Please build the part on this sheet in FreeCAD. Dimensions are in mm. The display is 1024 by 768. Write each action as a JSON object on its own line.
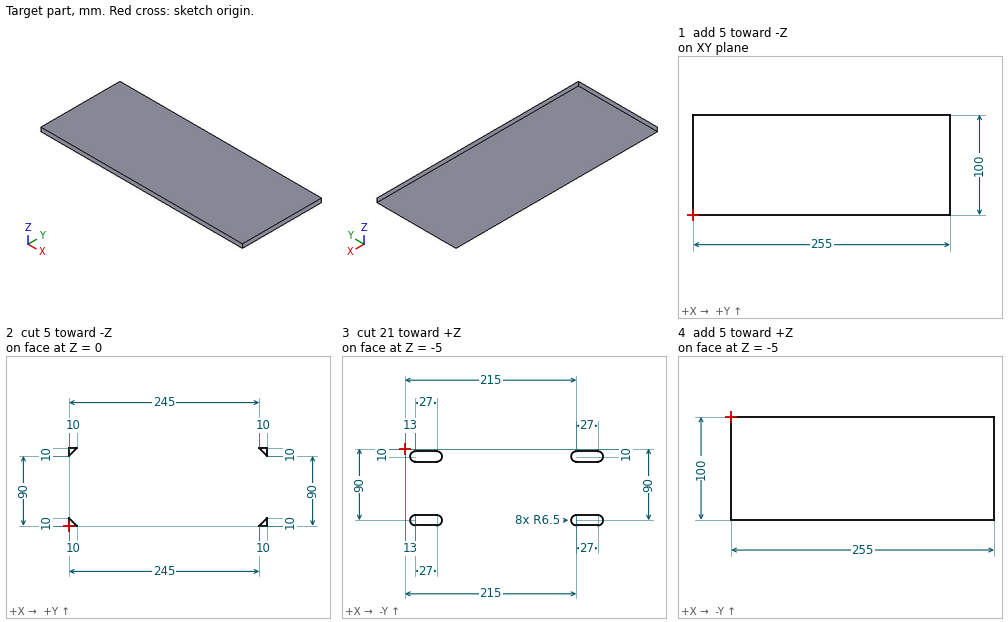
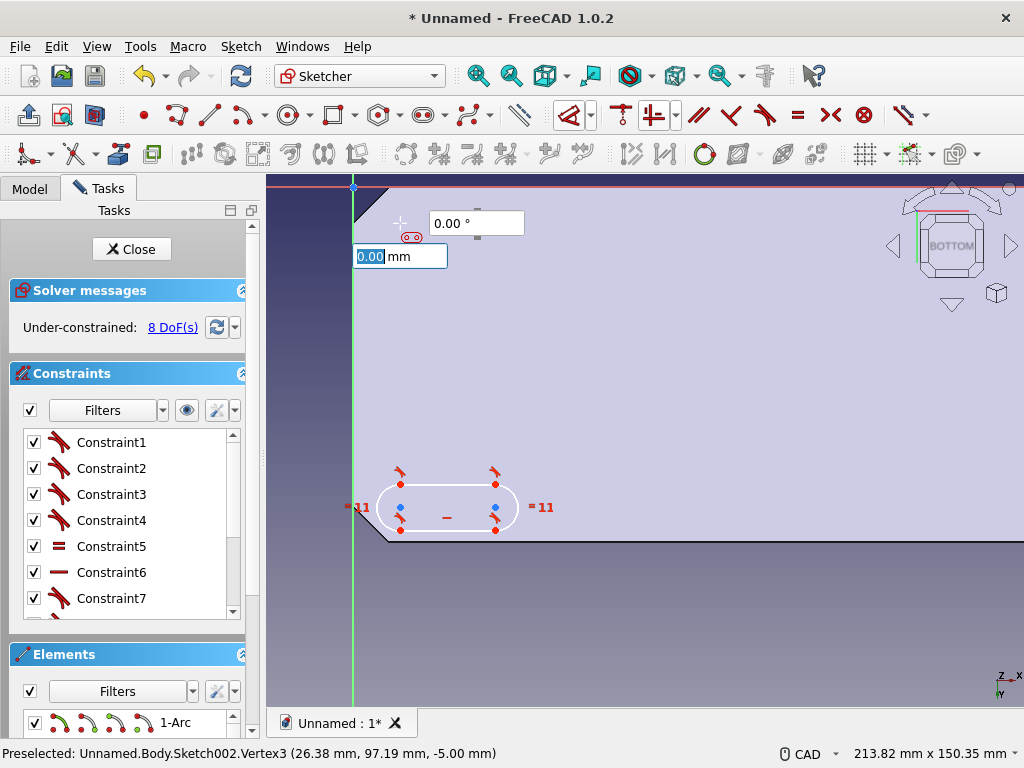
{"action": "left_click", "coordinate": [495, 223]}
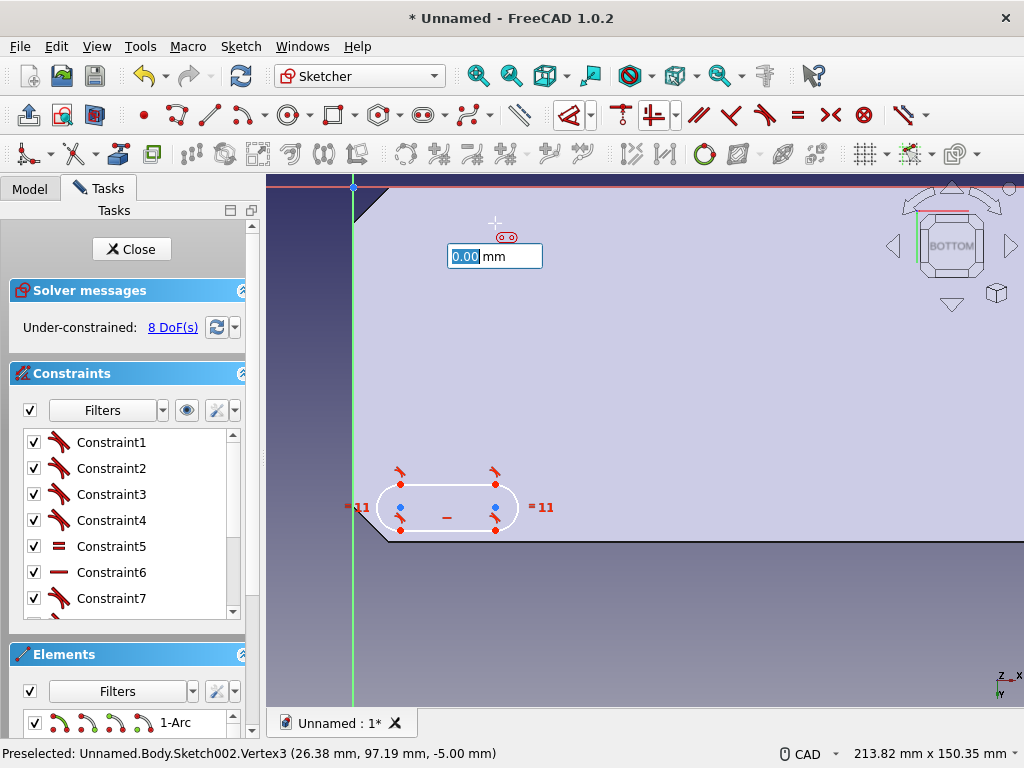
{"action": "left_click", "coordinate": [447, 246]}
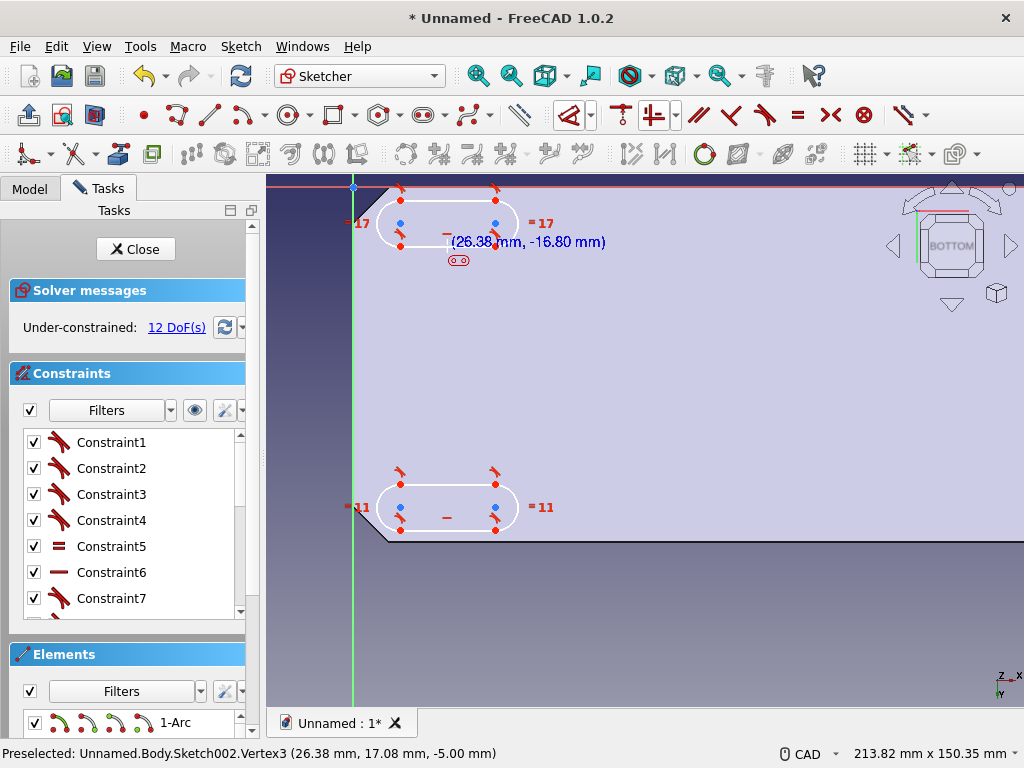
{"action": "scroll", "coordinate": [399, 507], "scroll_direction": "down", "scroll_amount": 4}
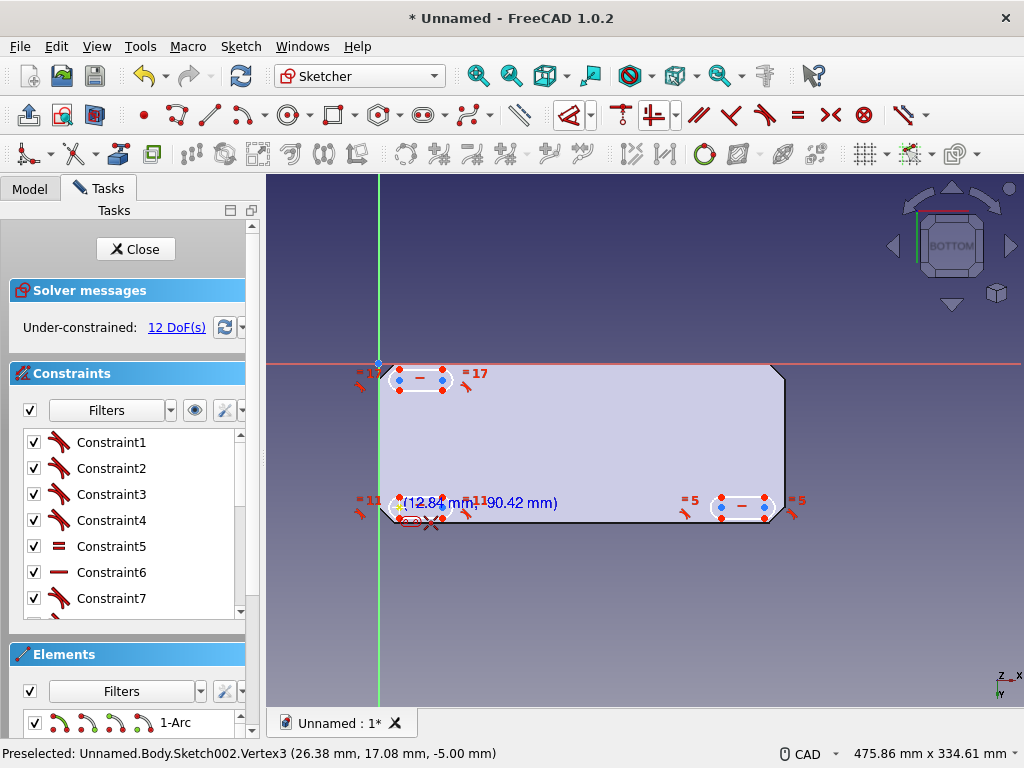
{"action": "scroll", "coordinate": [721, 380], "scroll_direction": "up", "scroll_amount": 4}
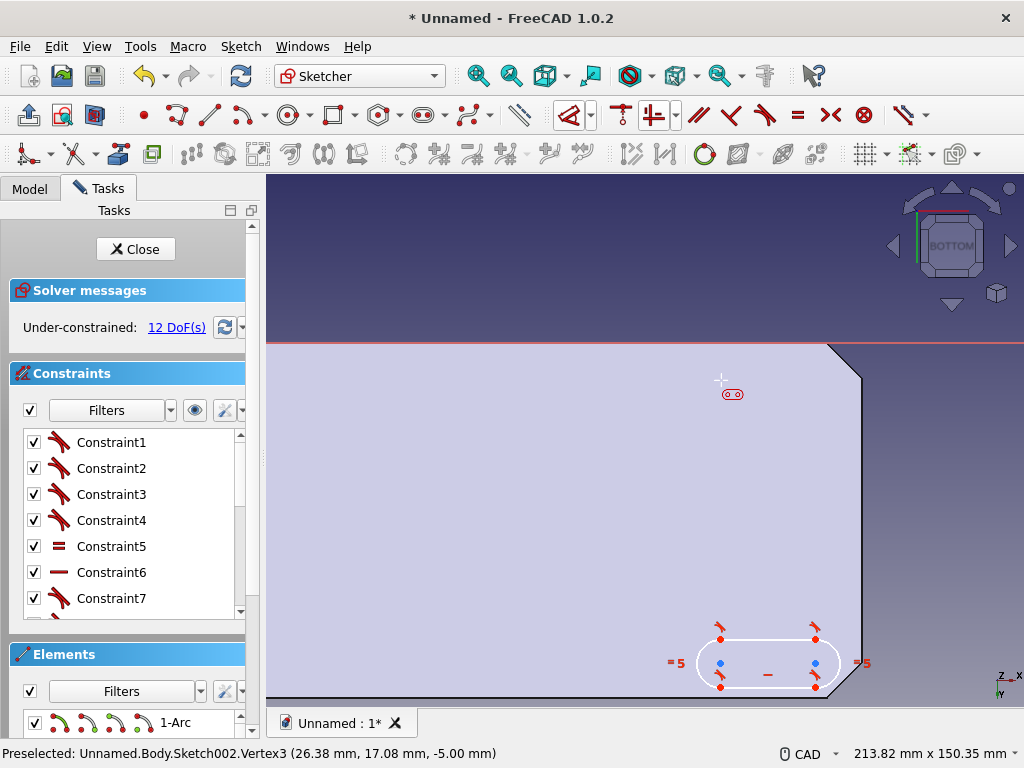
{"action": "left_click", "coordinate": [721, 379]}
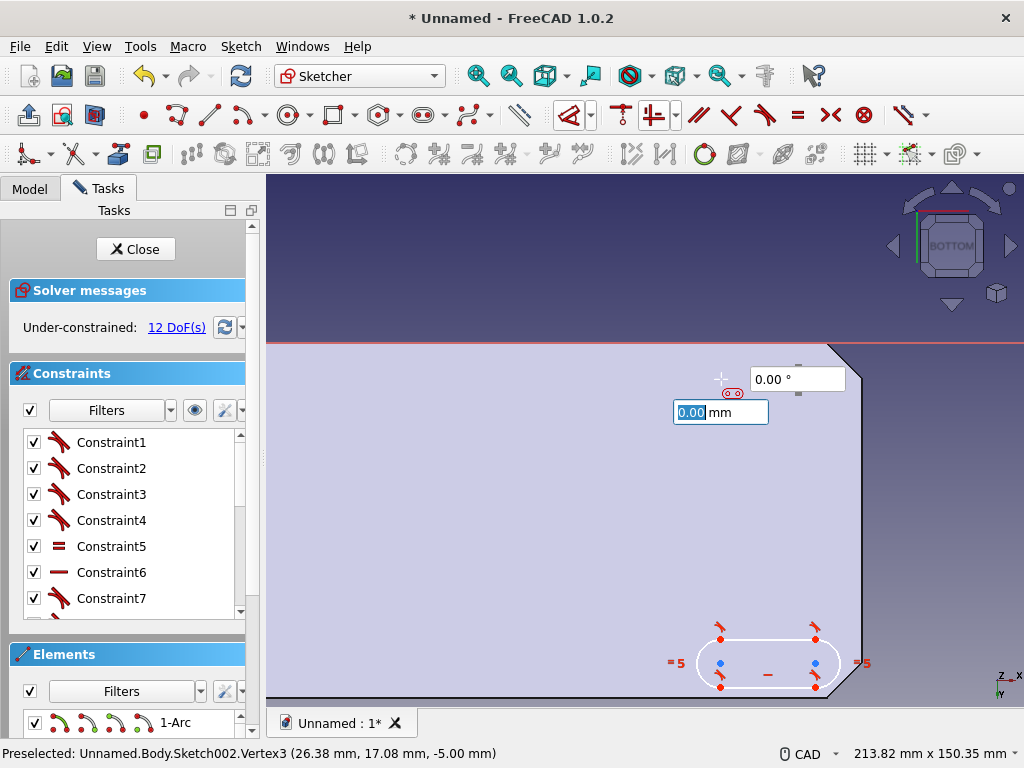
{"action": "left_click", "coordinate": [816, 379]}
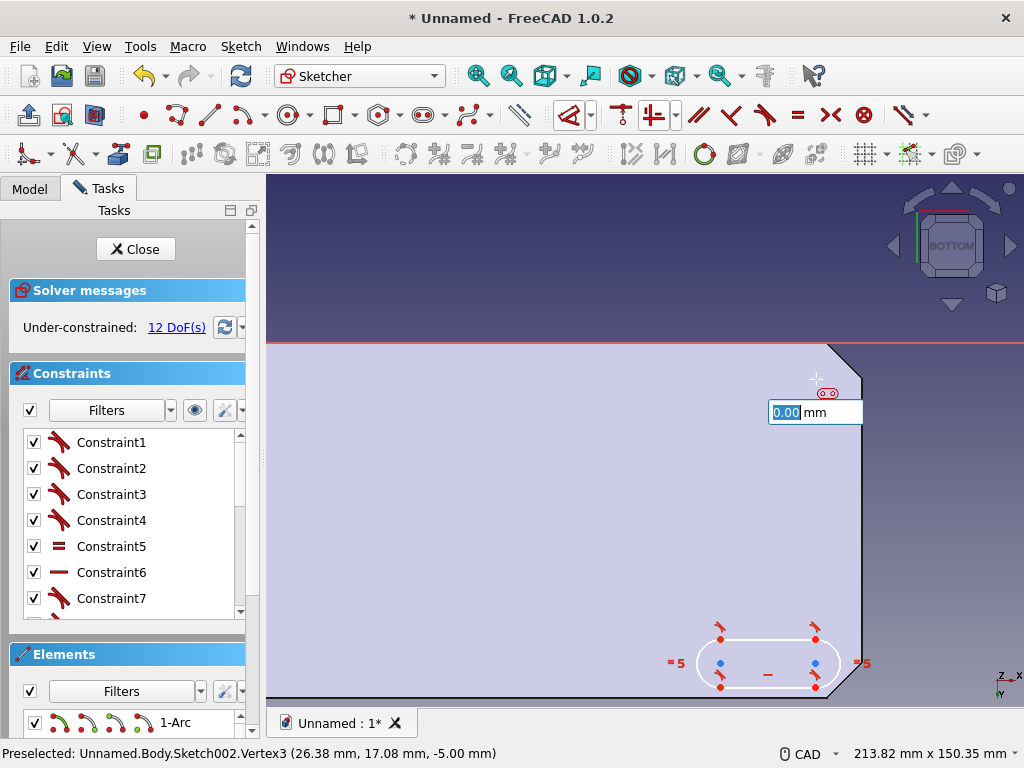
{"action": "left_click", "coordinate": [768, 402]}
{"action": "key", "text": "Escape"}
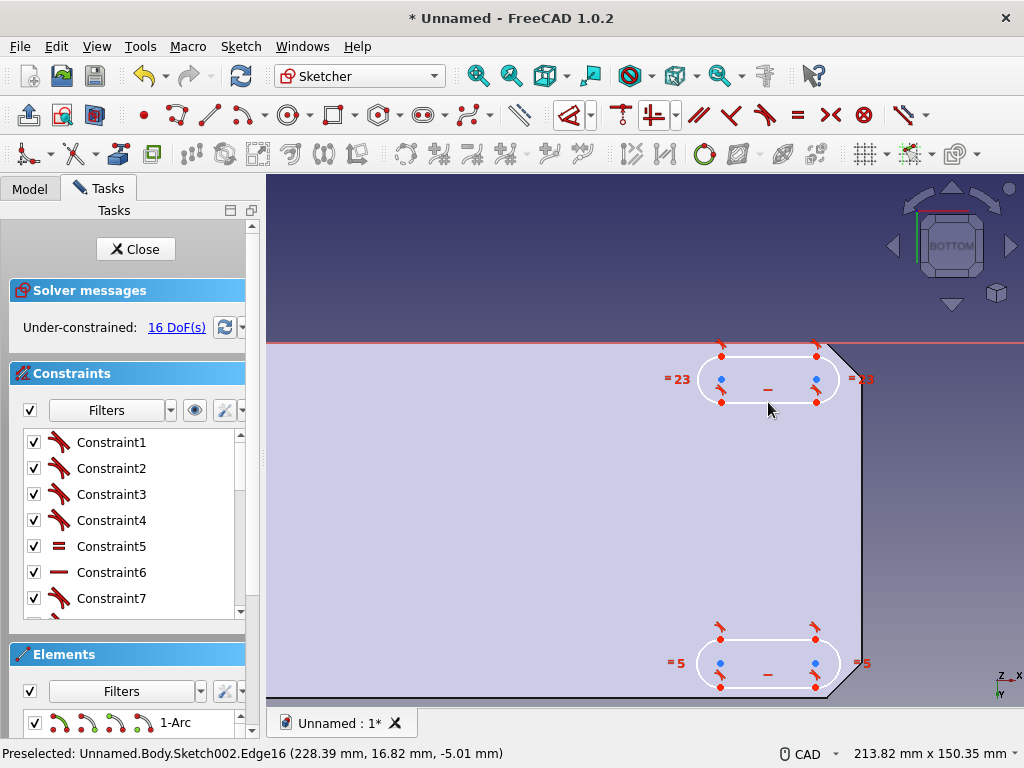
{"action": "left_click", "coordinate": [702, 650]}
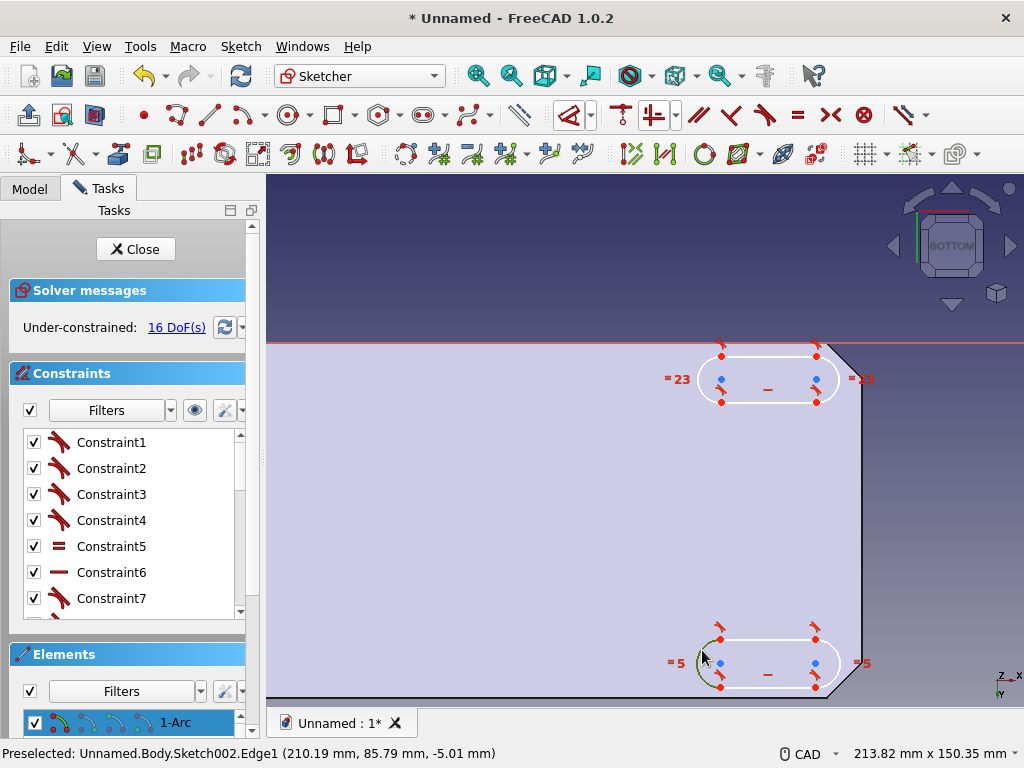
{"action": "scroll", "coordinate": [721, 380], "scroll_direction": "down", "scroll_amount": 4}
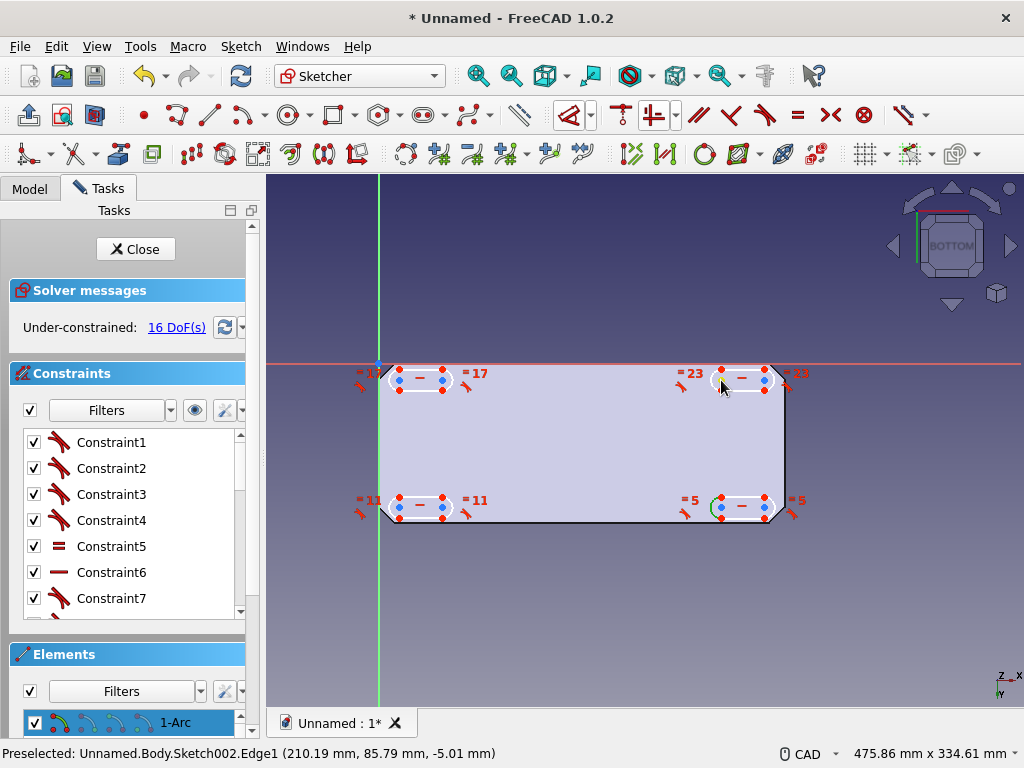
{"action": "scroll", "coordinate": [391, 502], "scroll_direction": "up", "scroll_amount": 2}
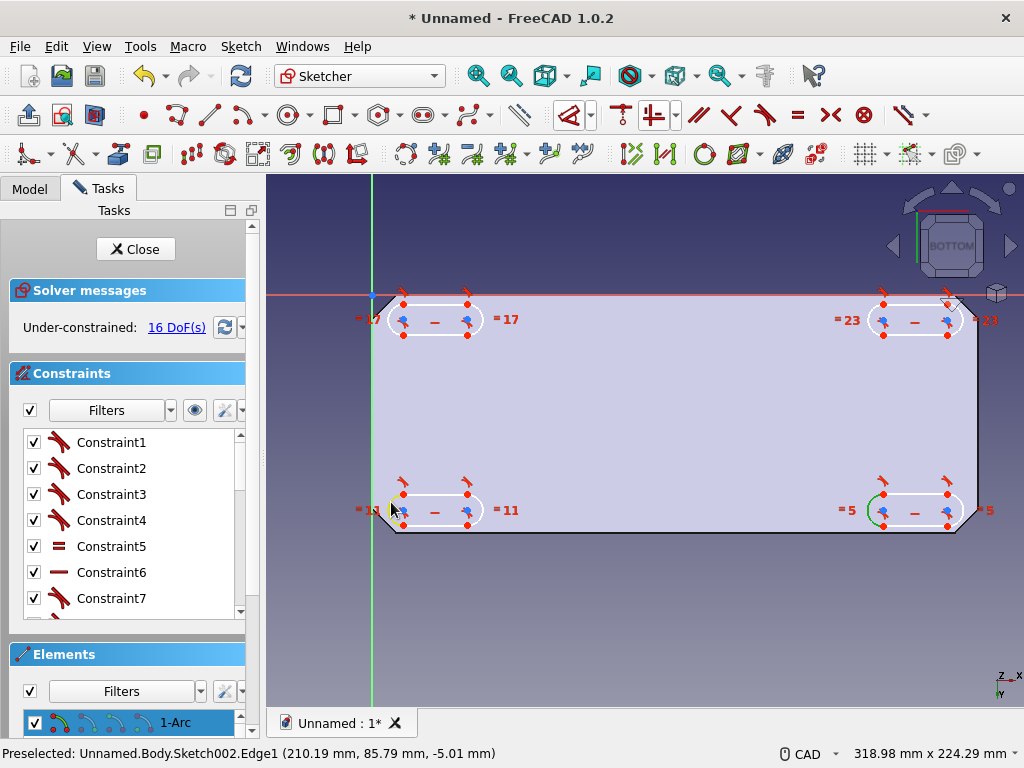
{"action": "left_click", "coordinate": [391, 501]}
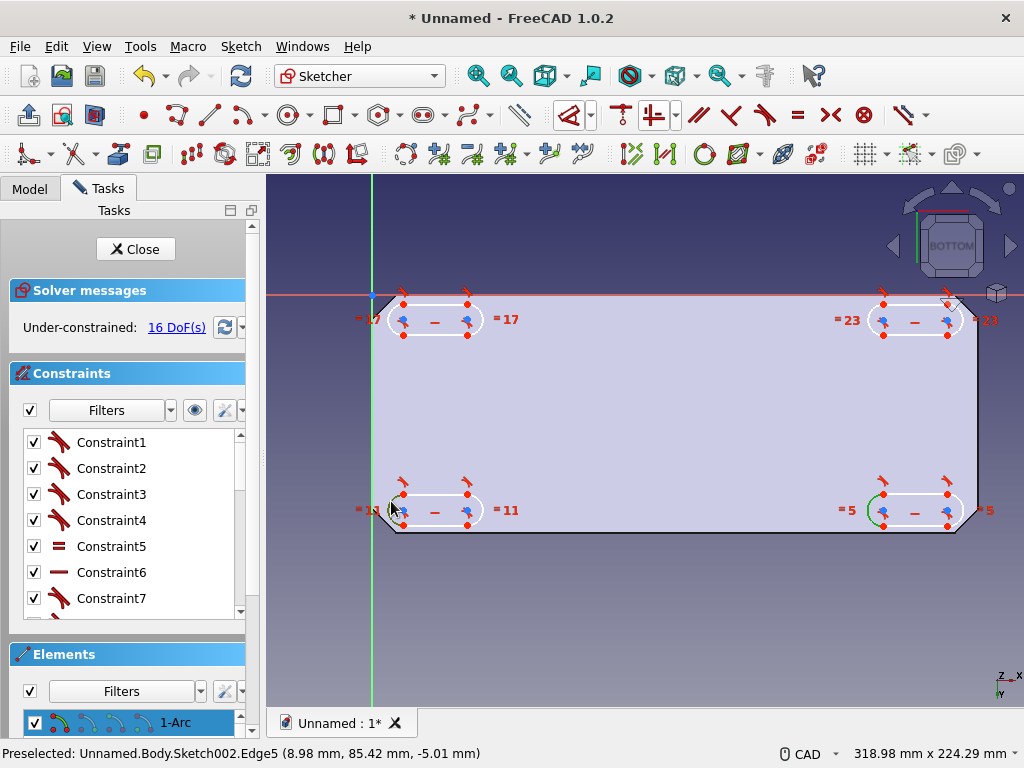
{"action": "left_click", "coordinate": [391, 311]}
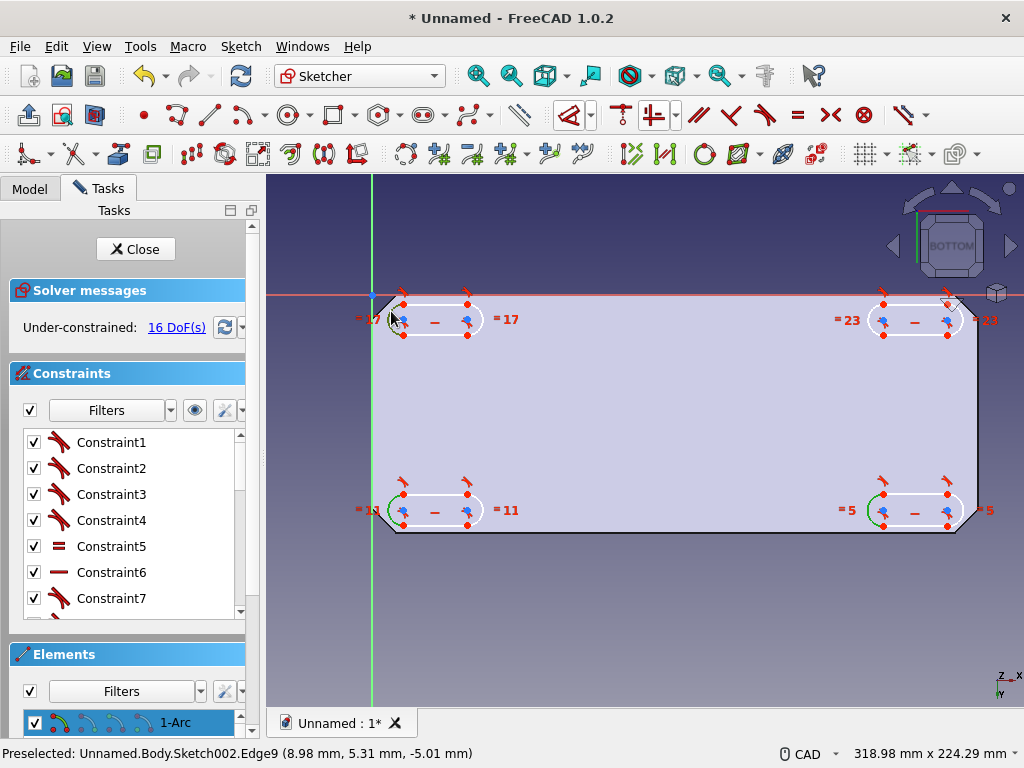
{"action": "scroll", "coordinate": [391, 502], "scroll_direction": "down", "scroll_amount": 2}